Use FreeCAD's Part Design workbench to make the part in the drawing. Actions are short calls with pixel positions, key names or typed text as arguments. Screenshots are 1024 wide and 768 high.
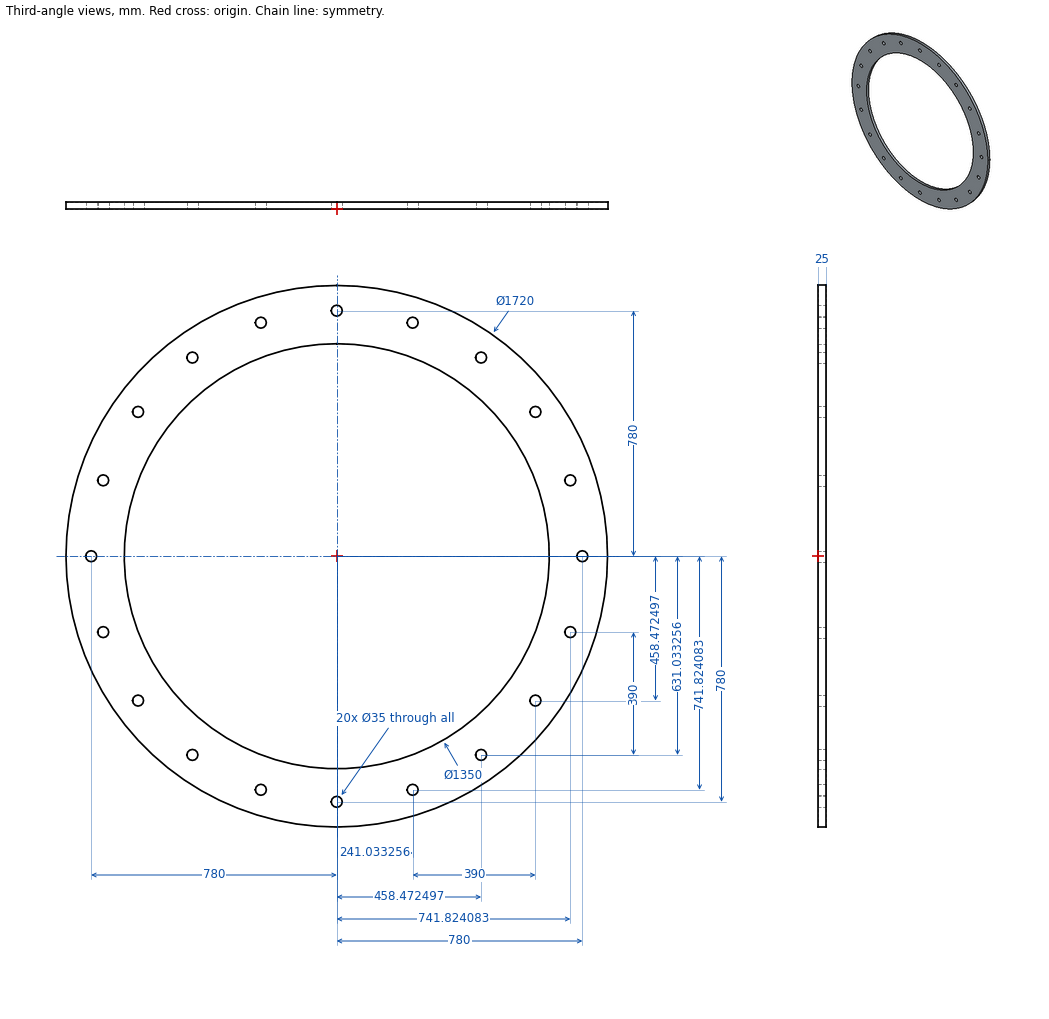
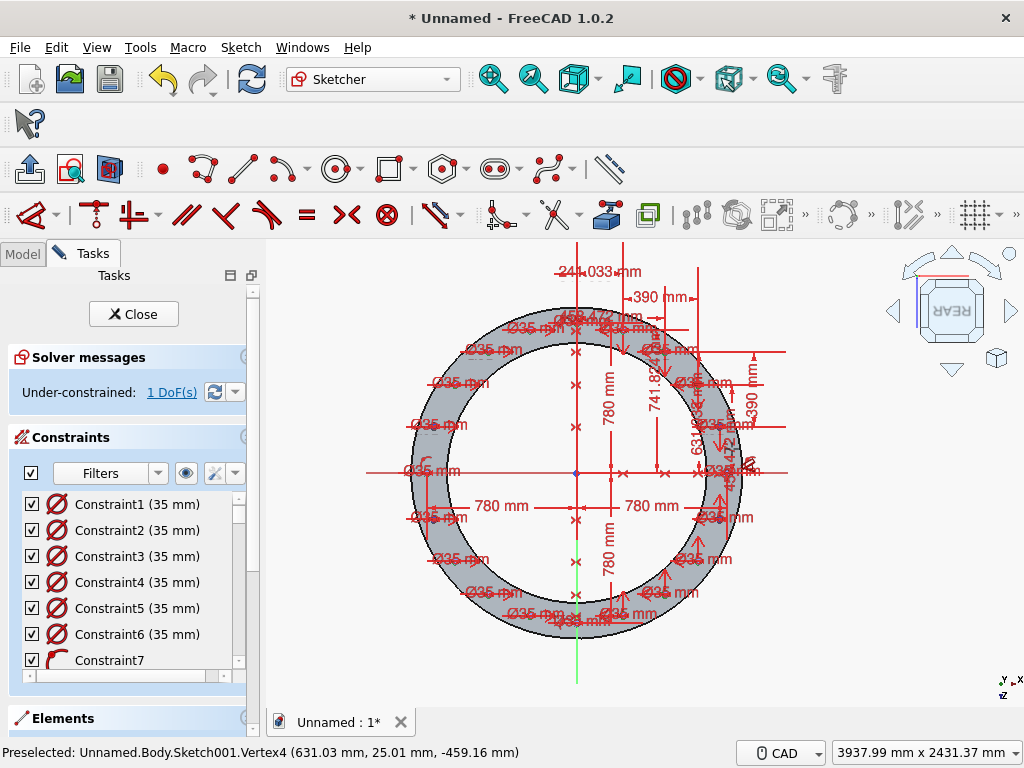
click(720, 427)
click(681, 531)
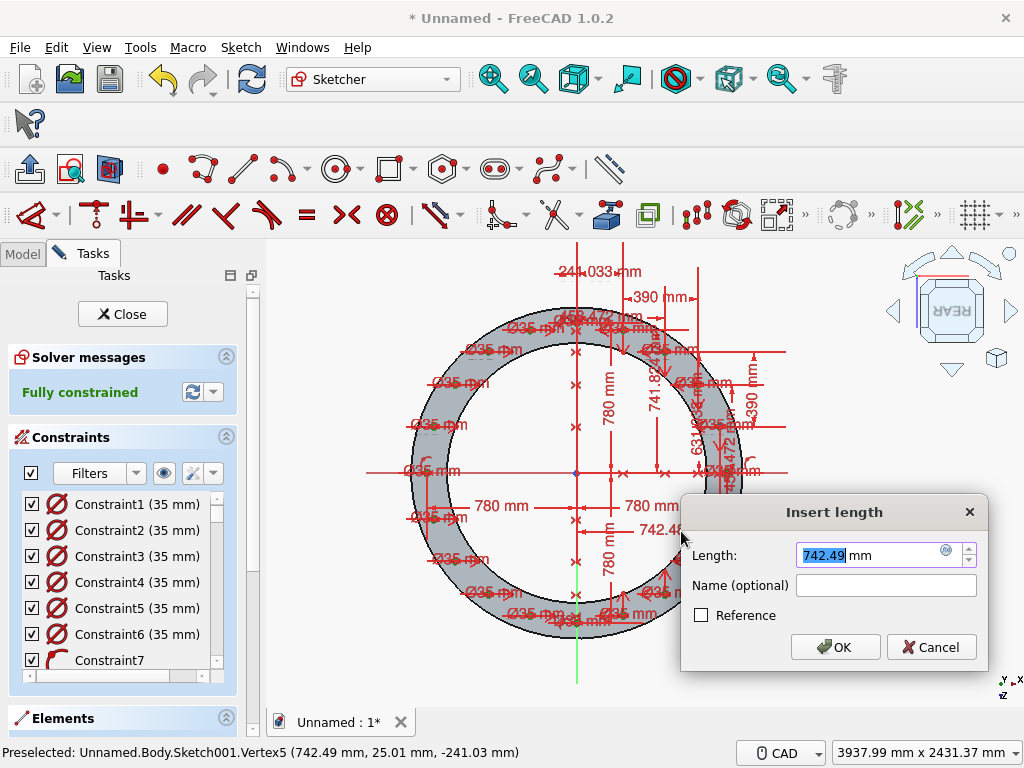
text(741.824083)
key(Return)
key(Escape)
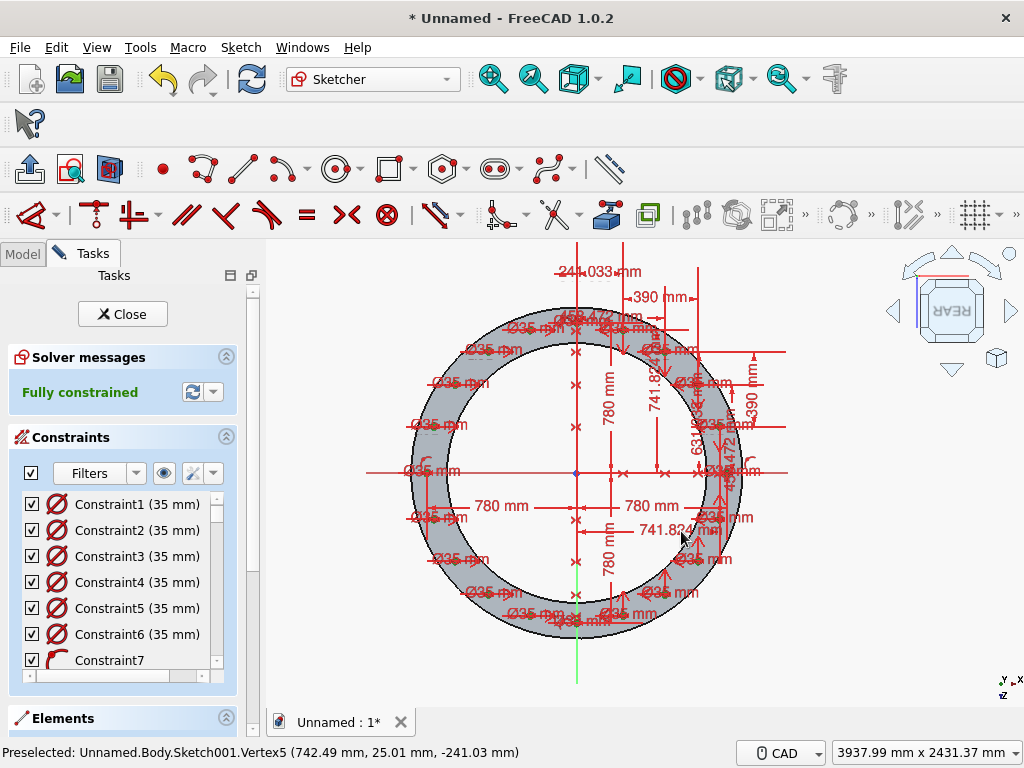
click(123, 314)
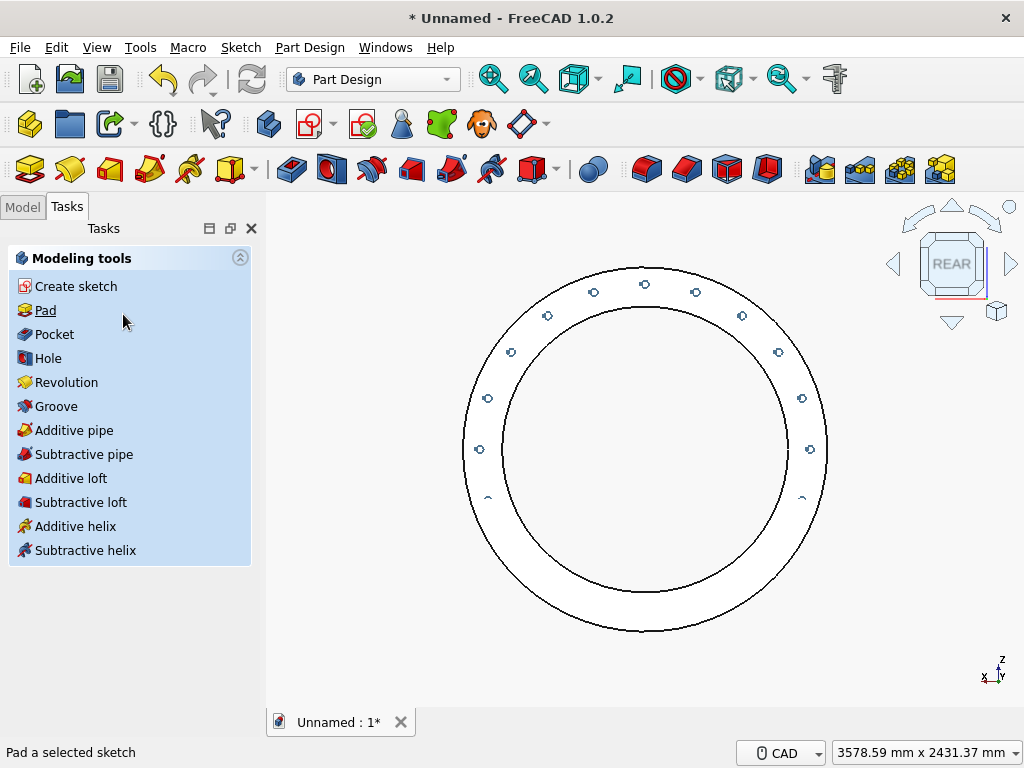
click(332, 170)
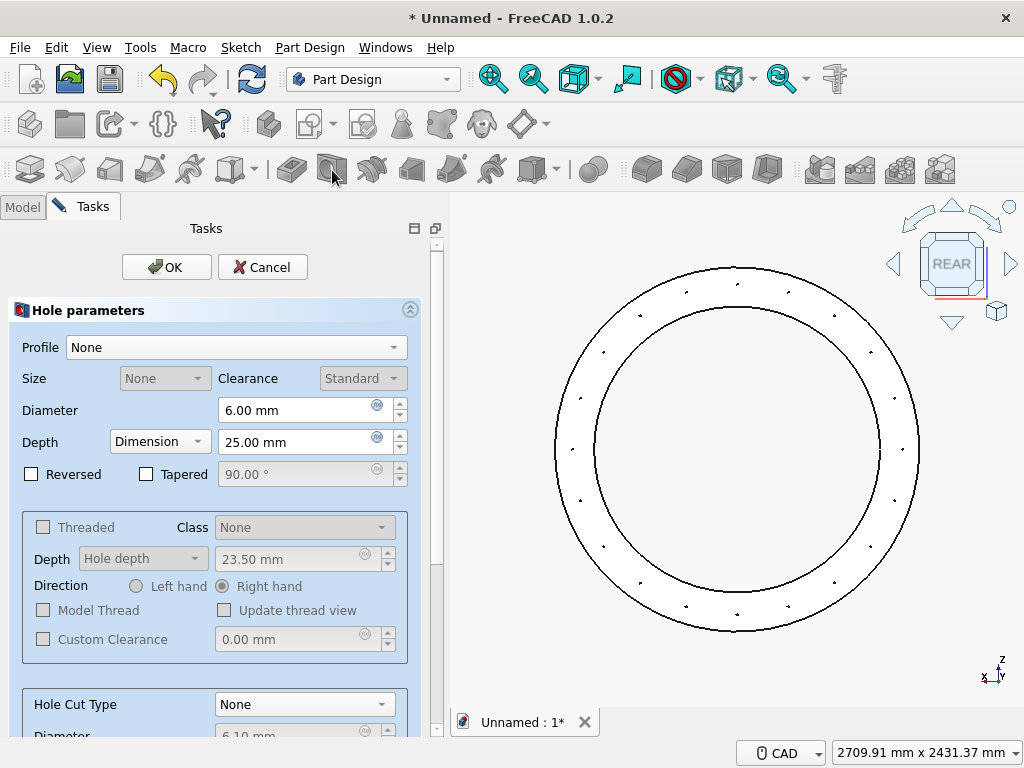
triple_click(305, 410)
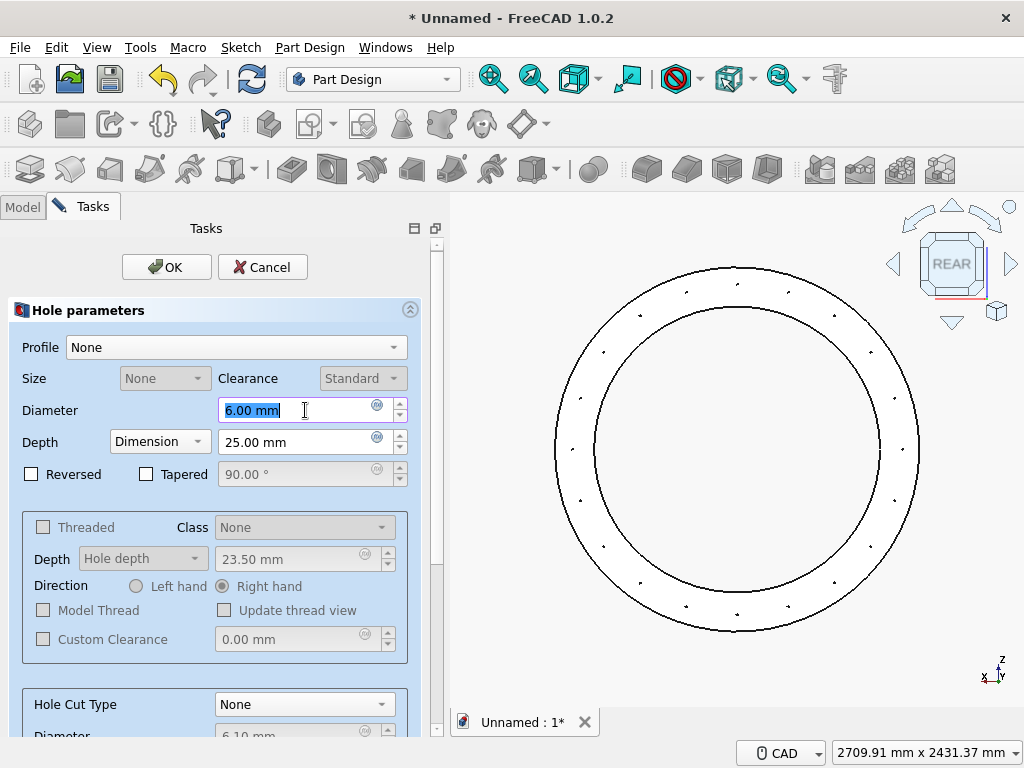
text(35)
key(Tab)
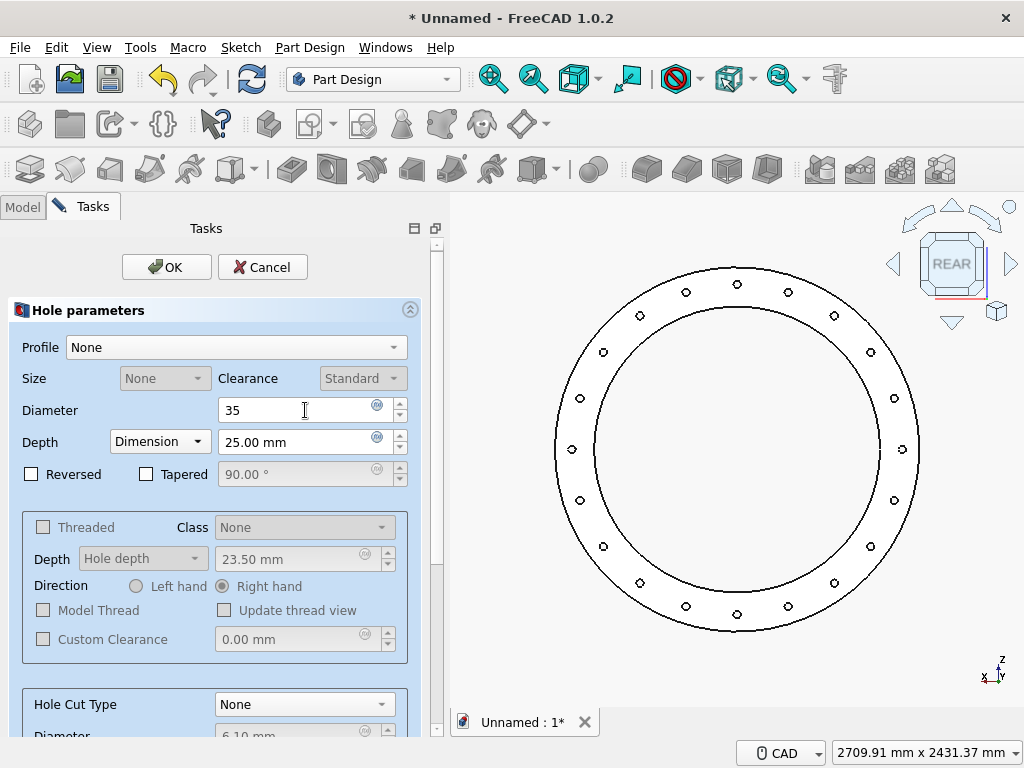
click(161, 442)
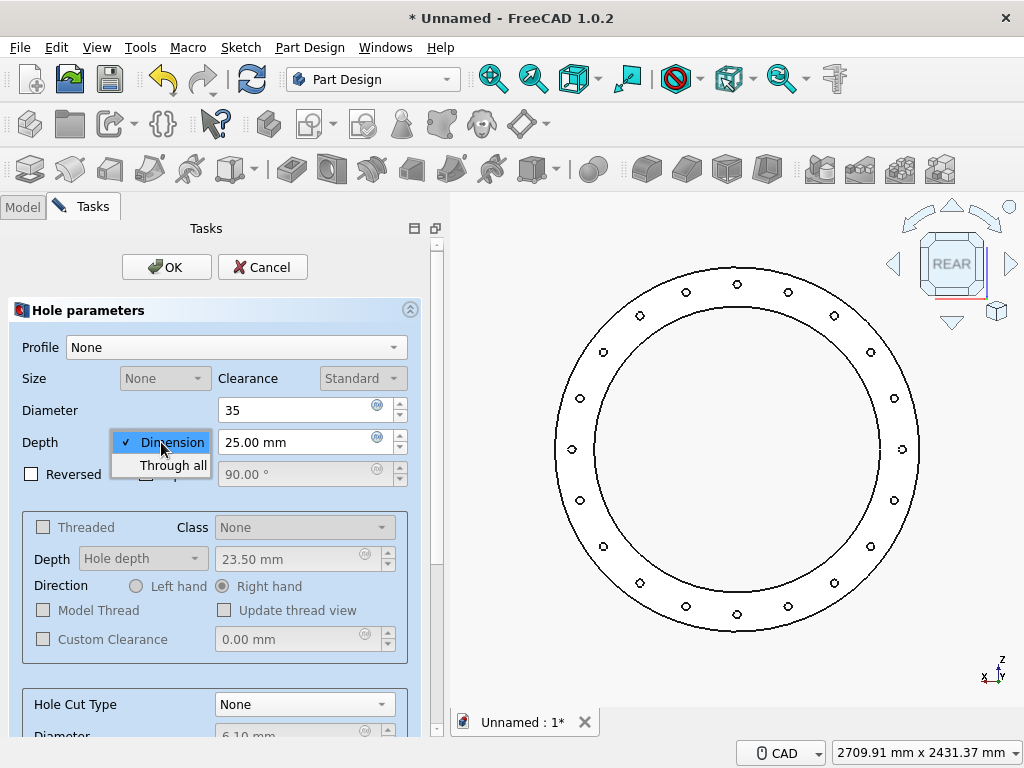
click(160, 466)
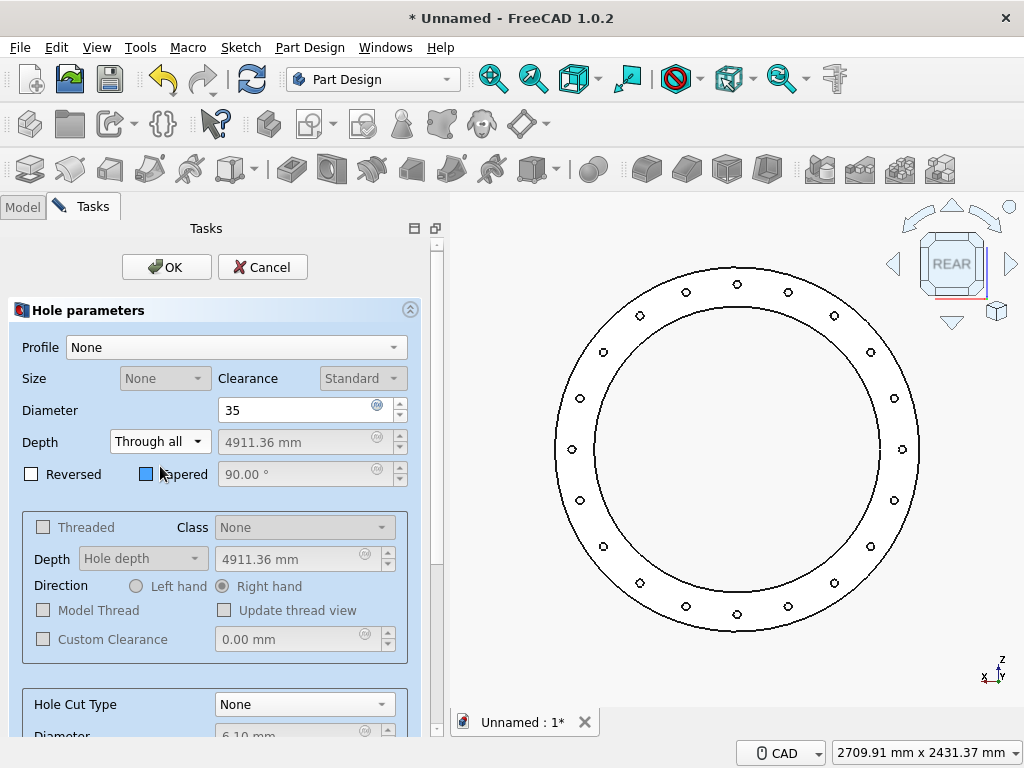
click(167, 267)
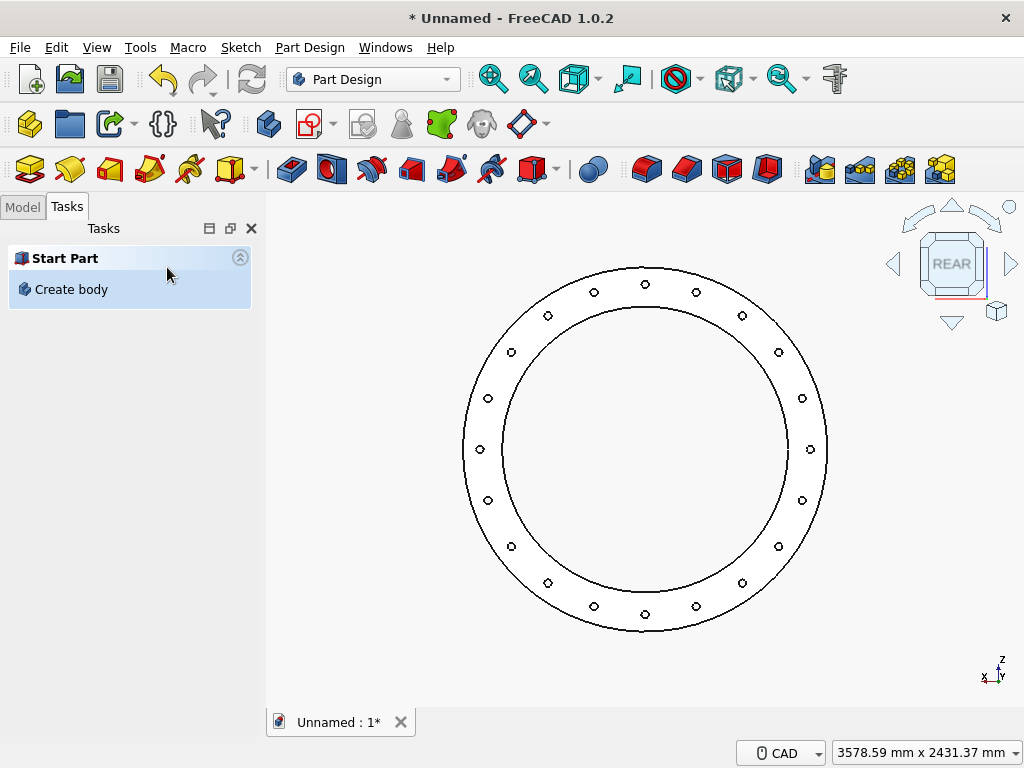
key(0)